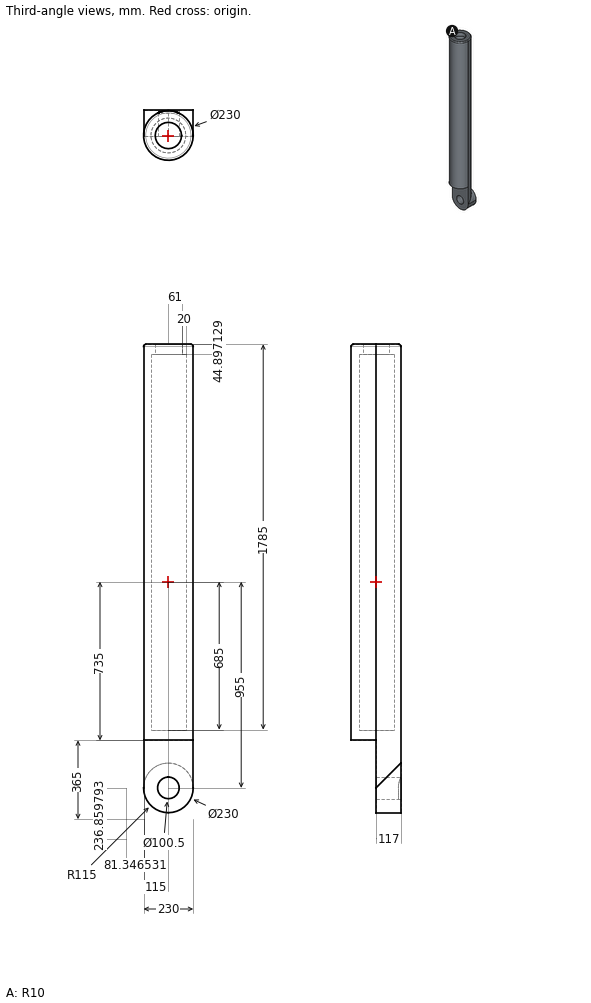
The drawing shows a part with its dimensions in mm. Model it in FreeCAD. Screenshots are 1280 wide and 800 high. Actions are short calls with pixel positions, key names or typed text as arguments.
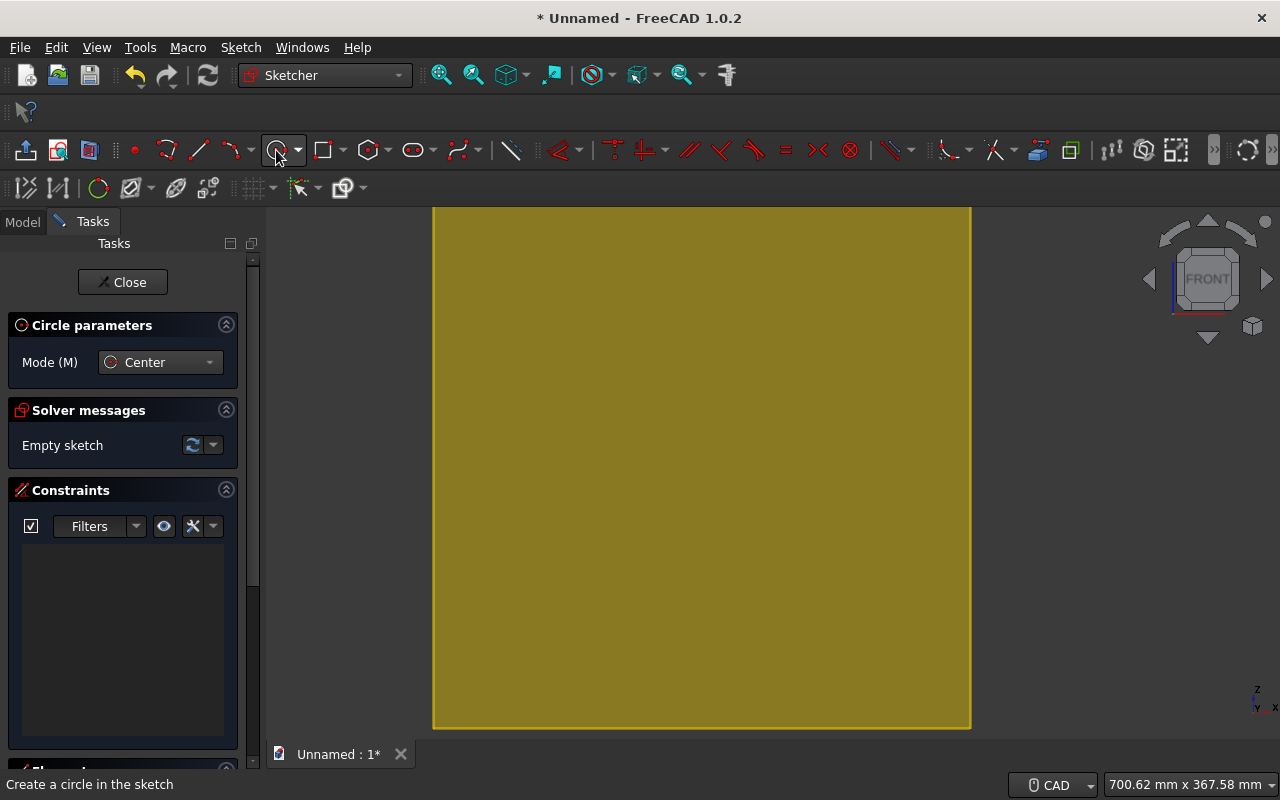
click(702, 460)
click(820, 342)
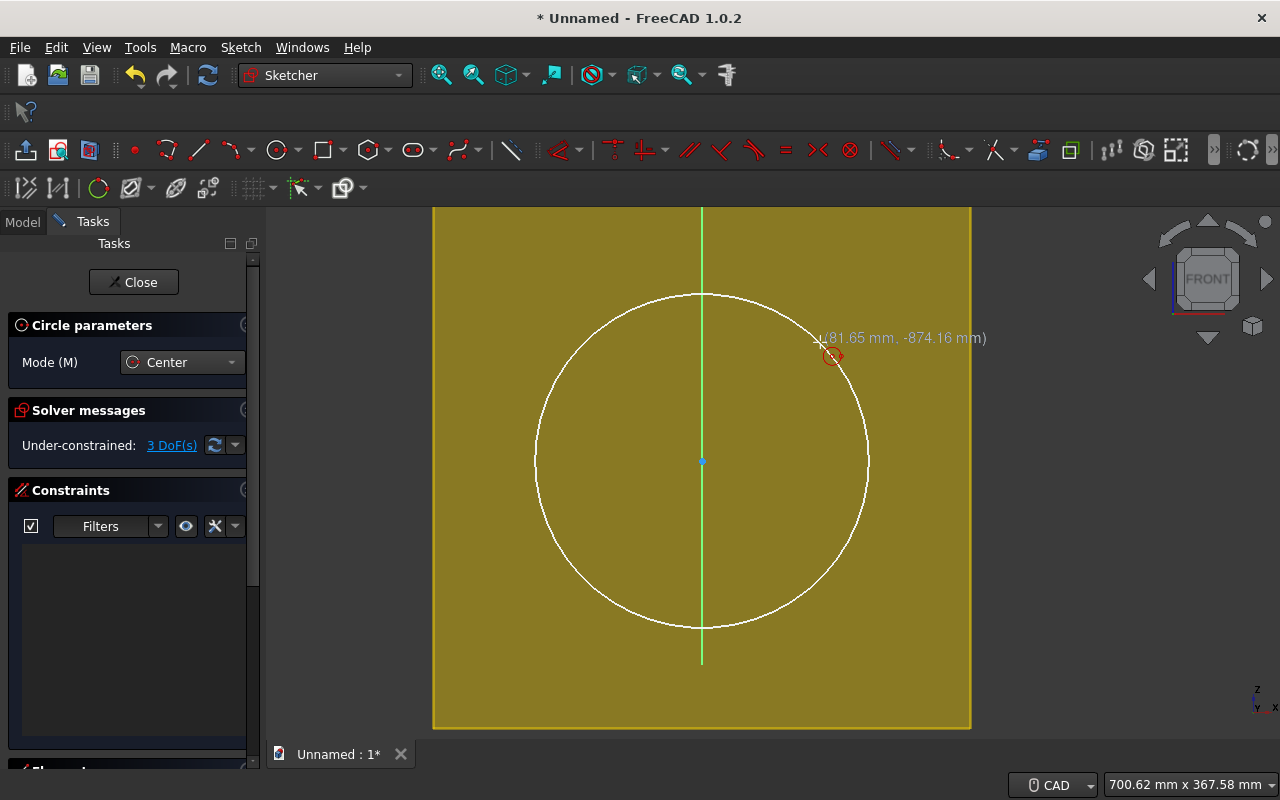
click(702, 461)
click(753, 409)
key(Escape)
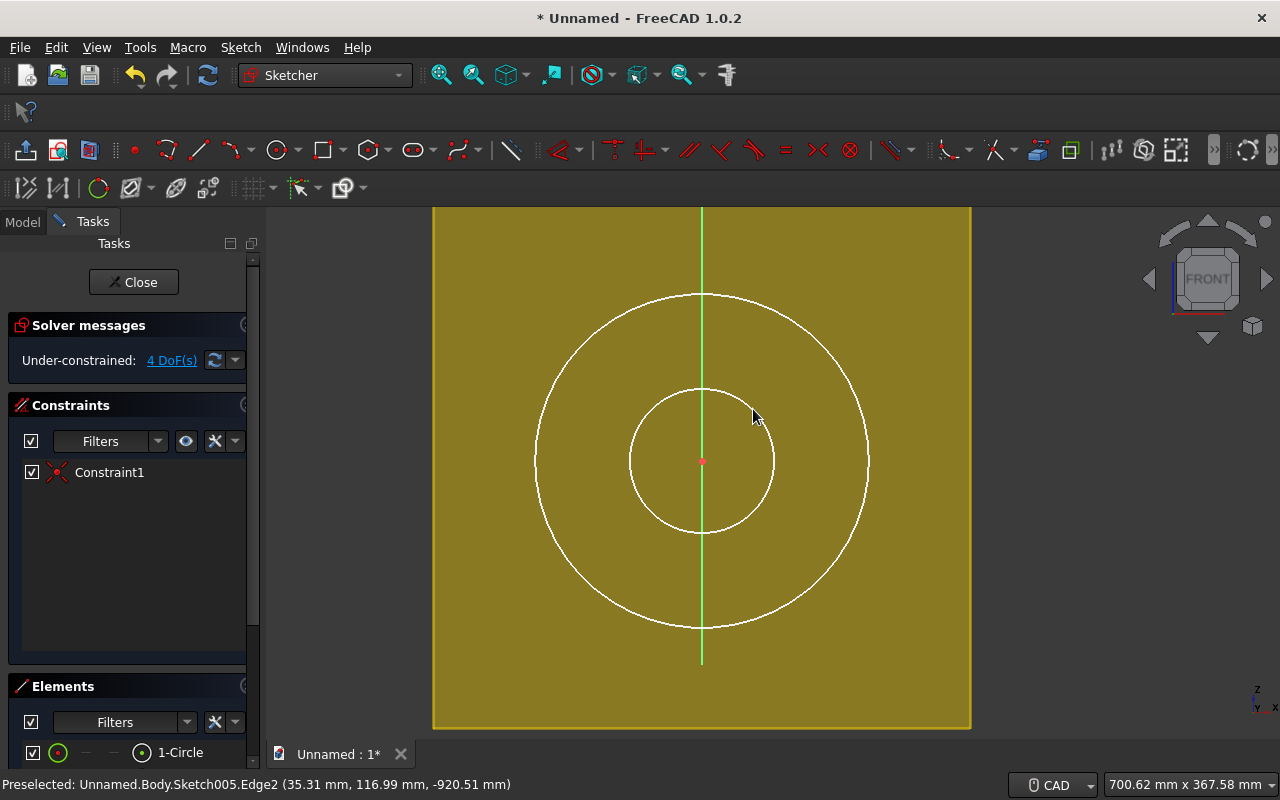
click(702, 461)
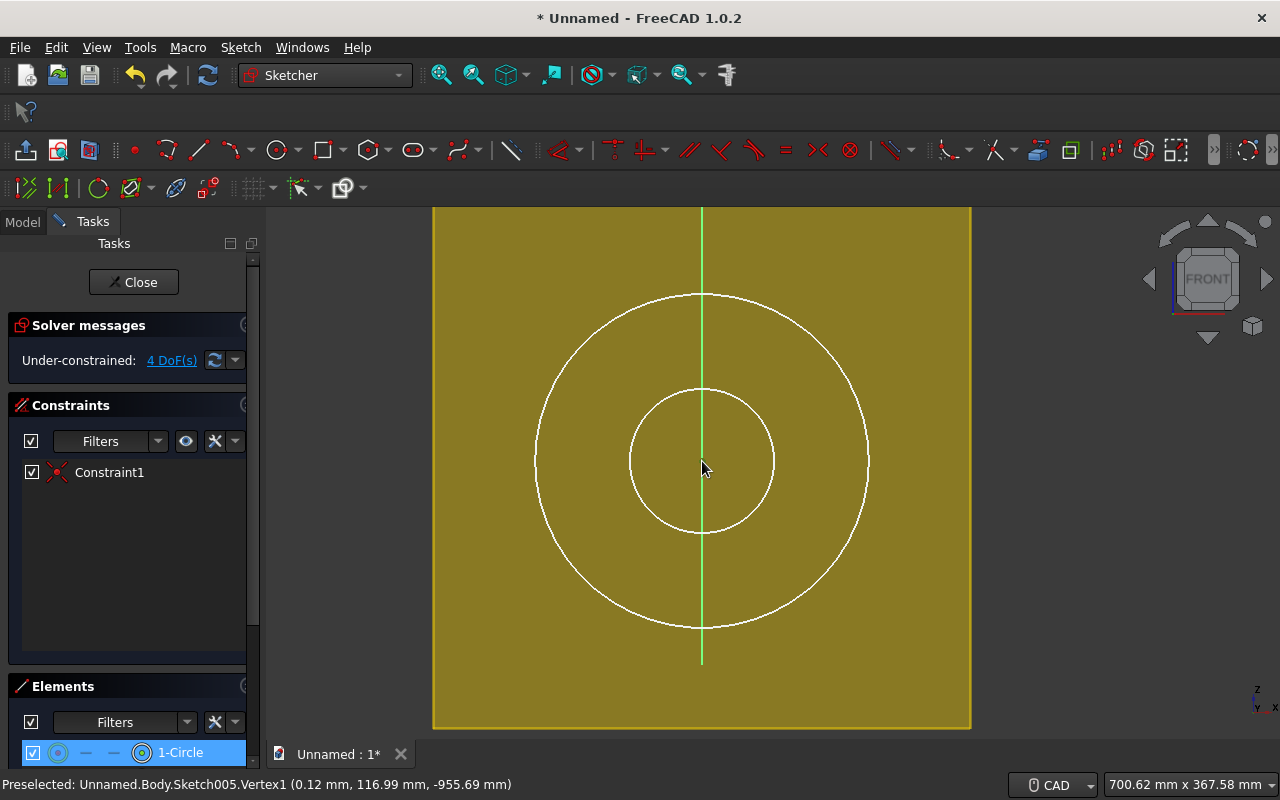
click(702, 575)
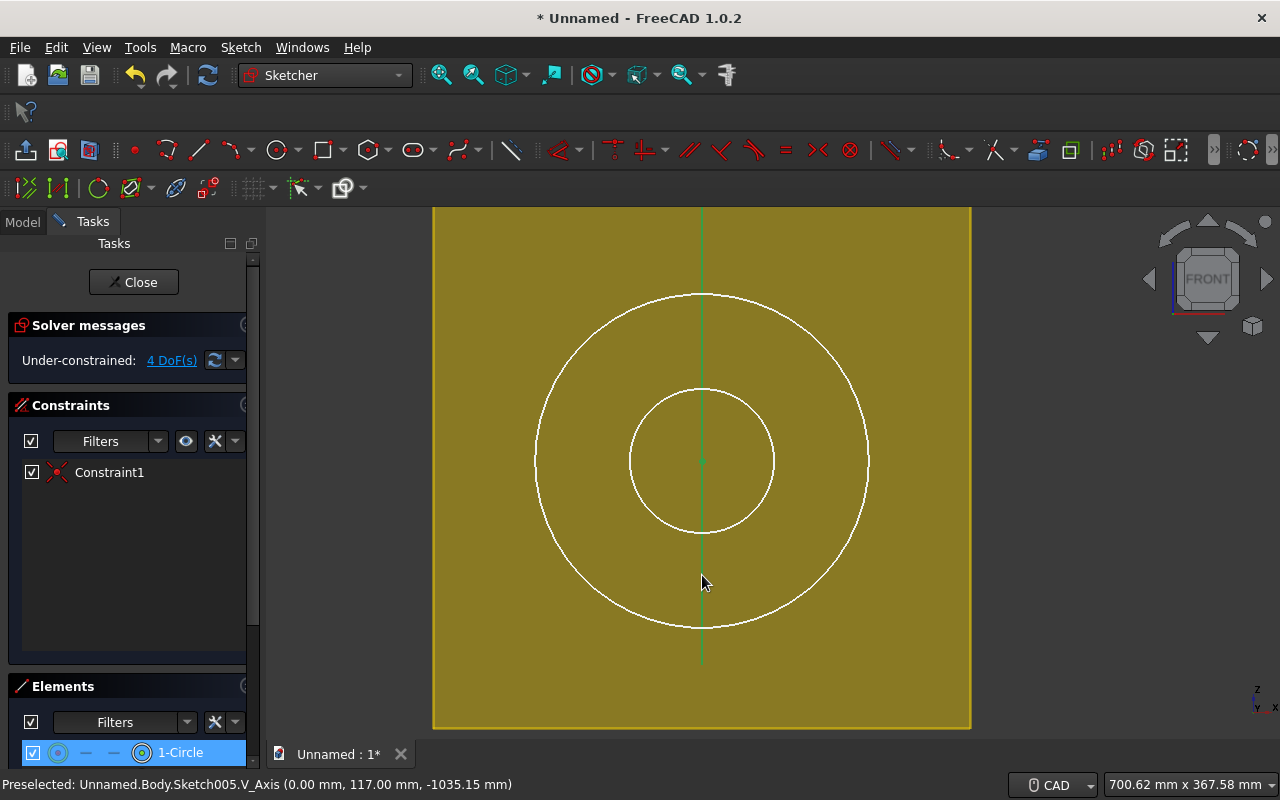
click(614, 150)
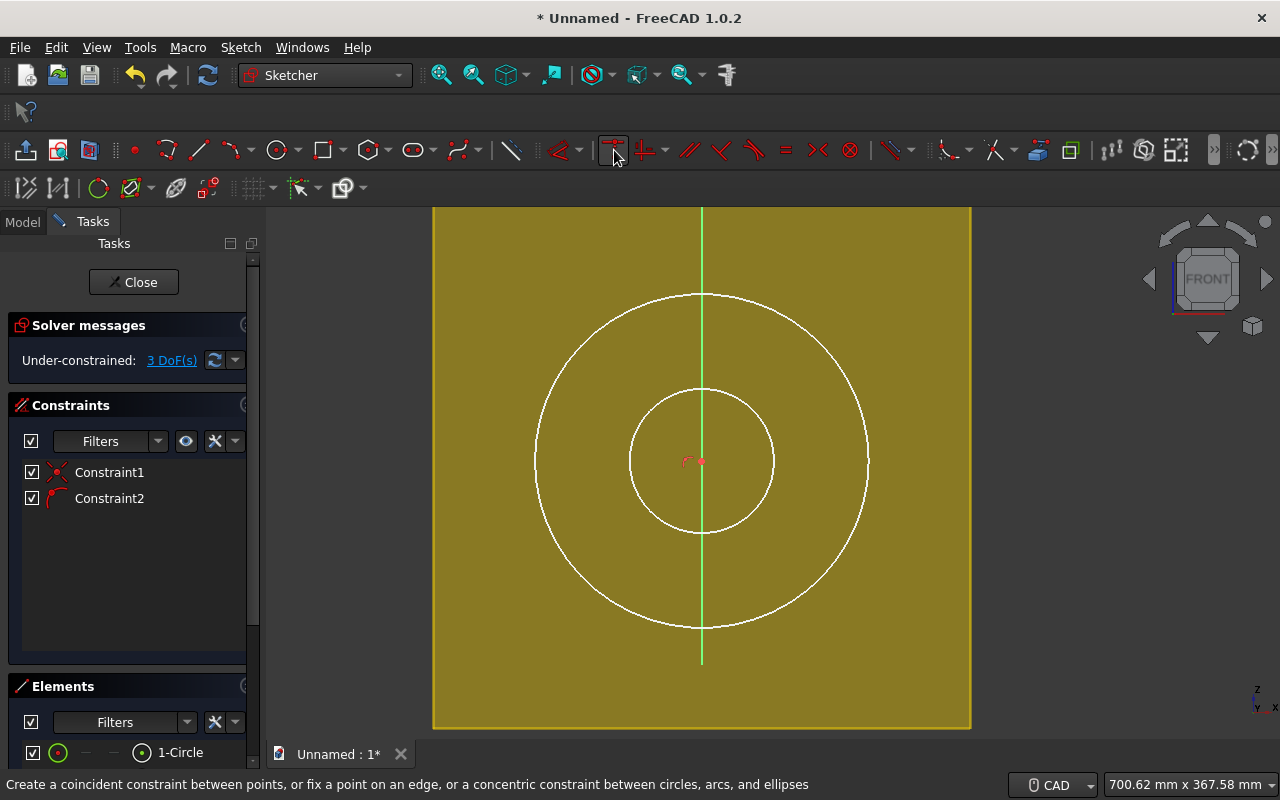
key(d)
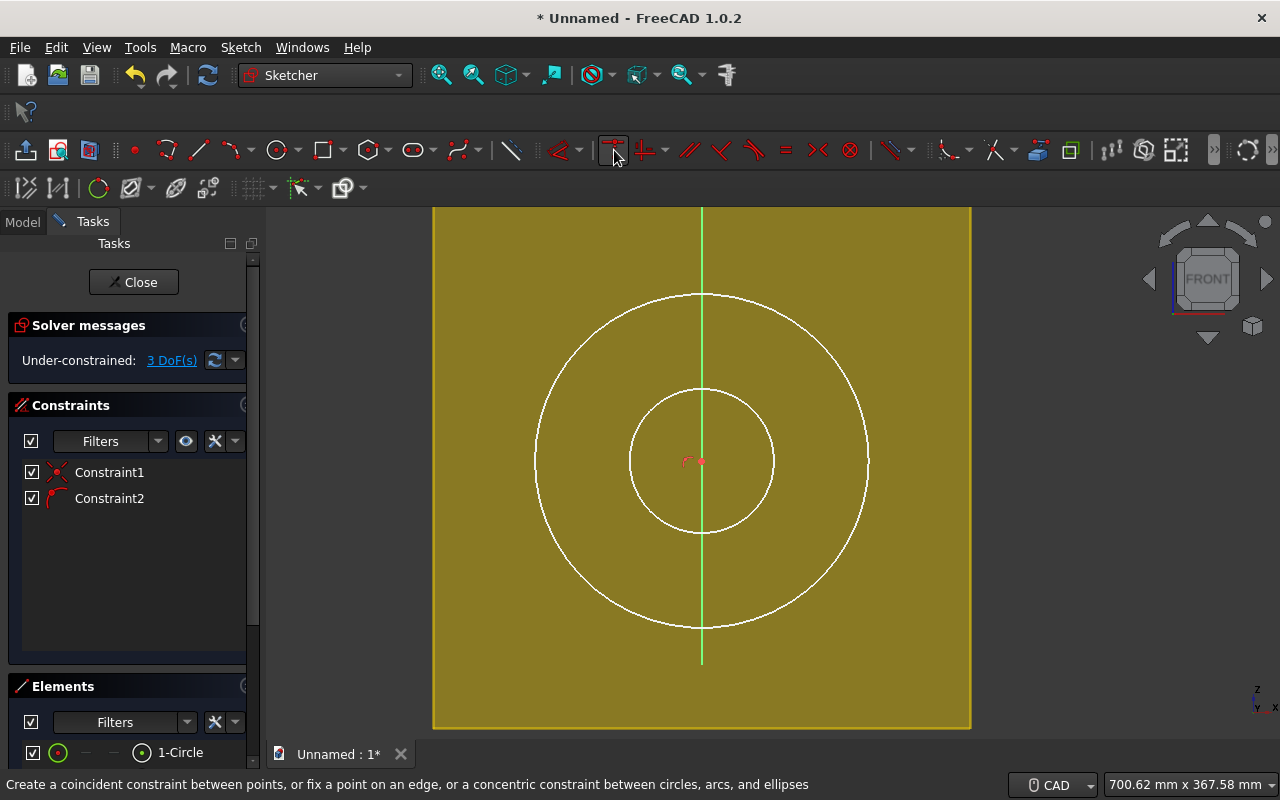
click(819, 343)
click(842, 320)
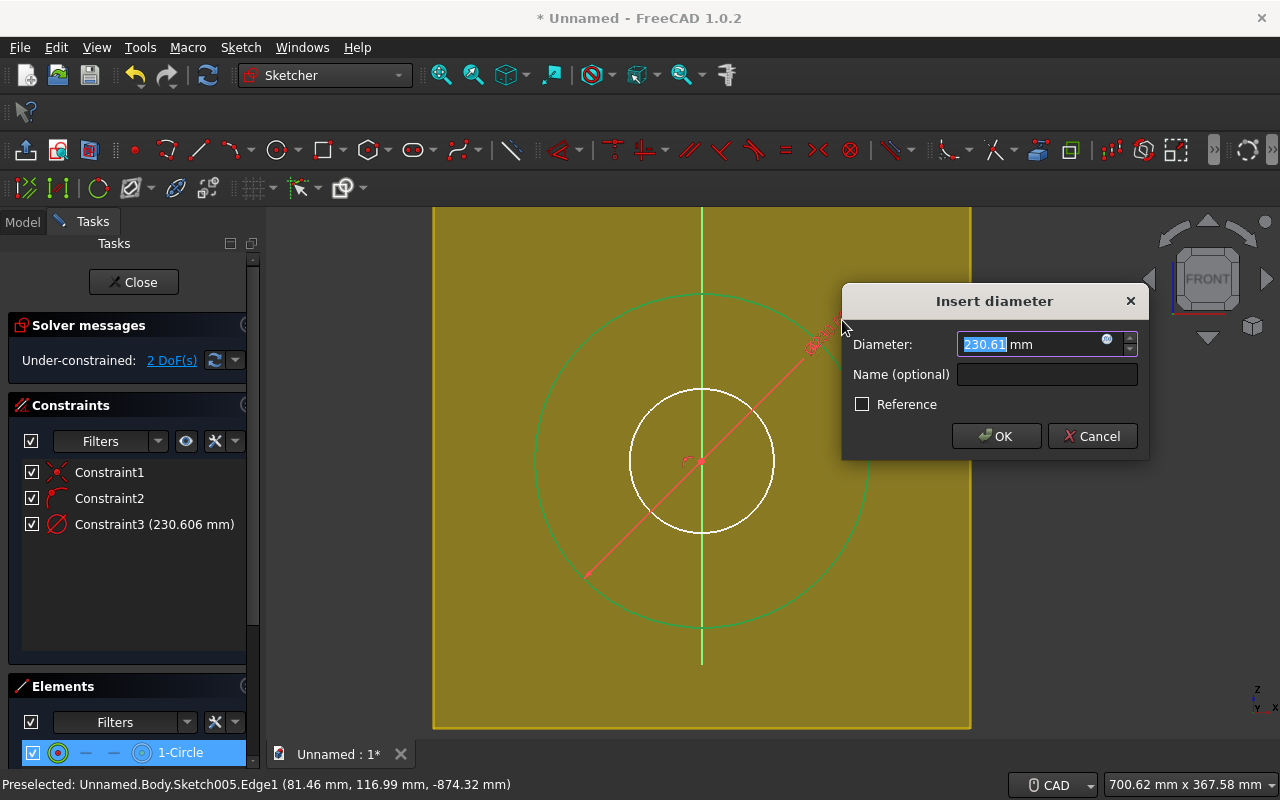
text(230)
key(Return)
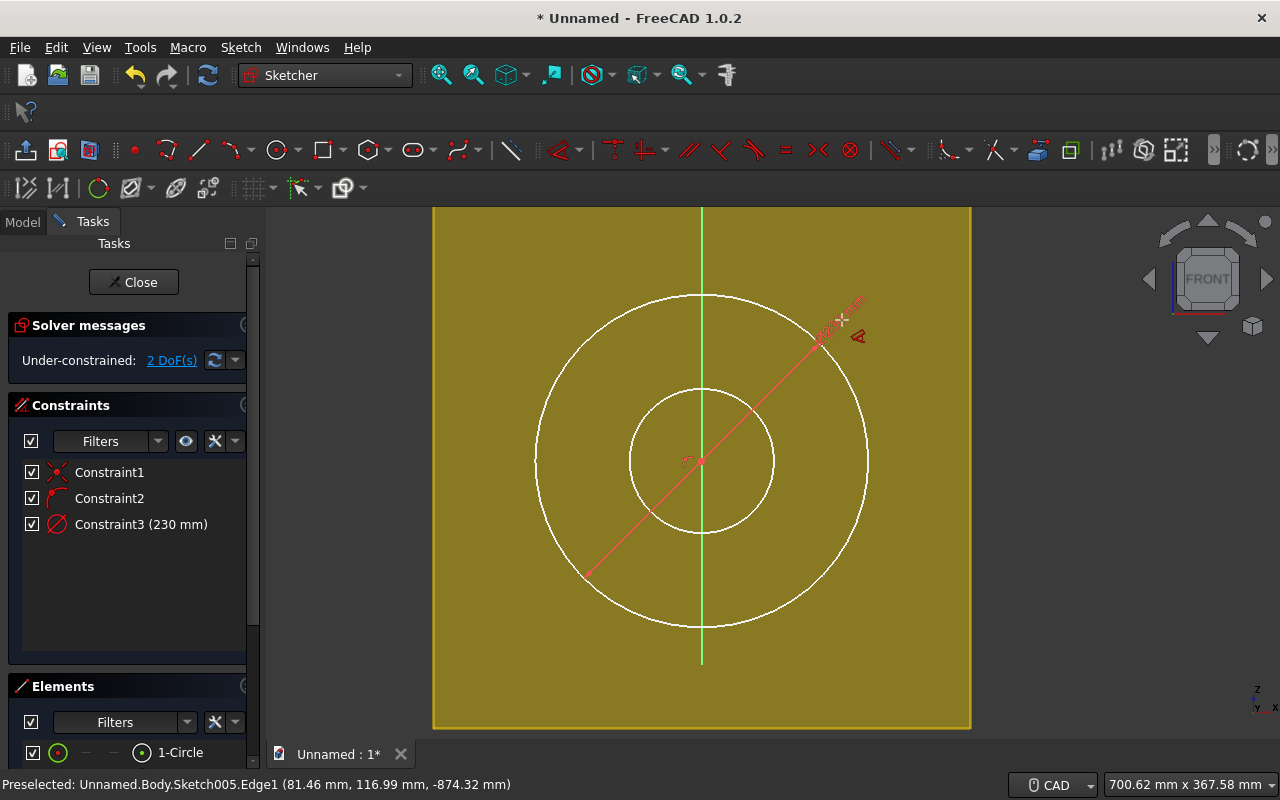
click(753, 410)
click(776, 387)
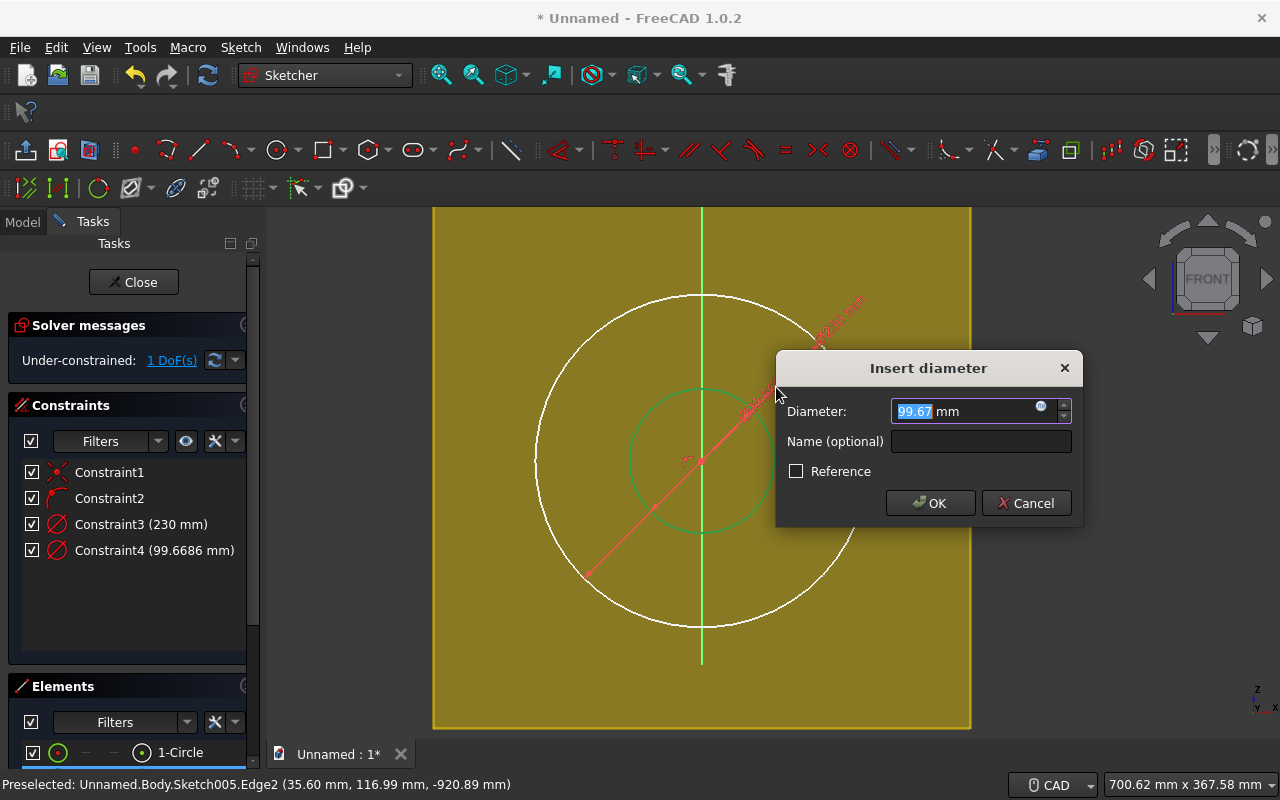
text(100.5)
key(Return)